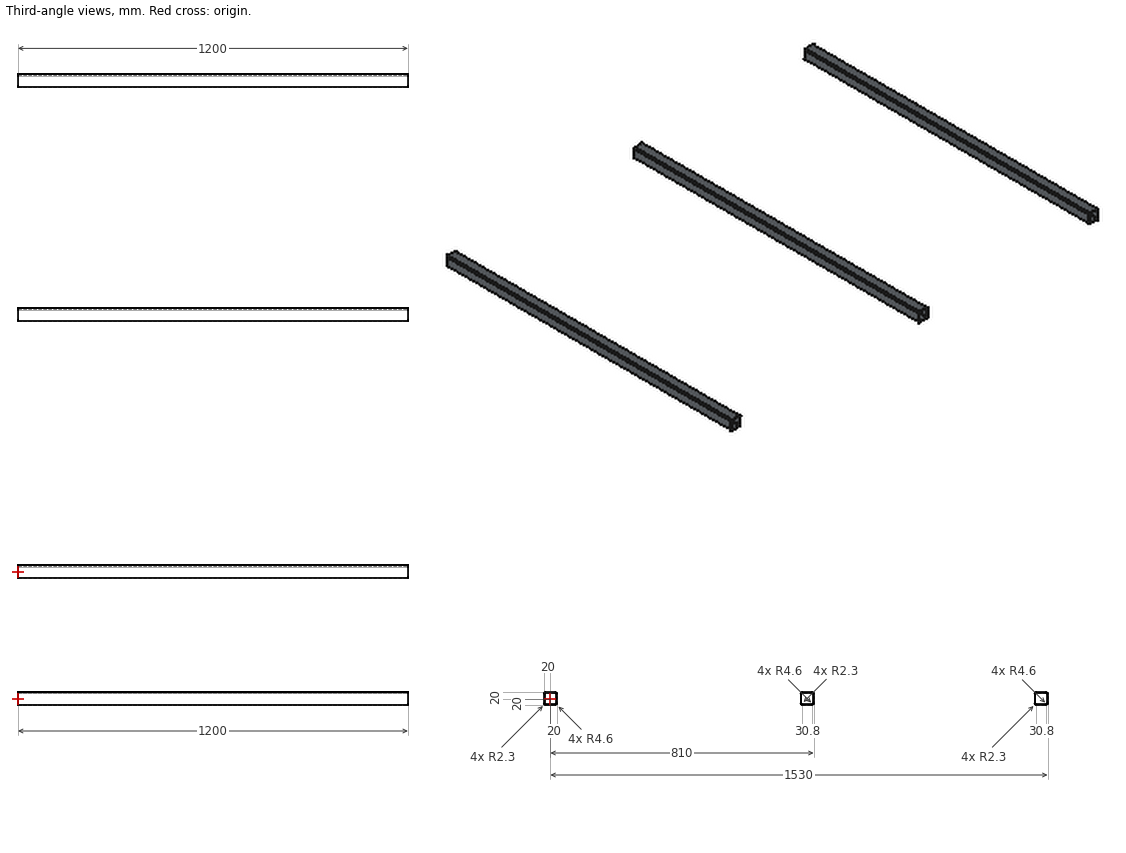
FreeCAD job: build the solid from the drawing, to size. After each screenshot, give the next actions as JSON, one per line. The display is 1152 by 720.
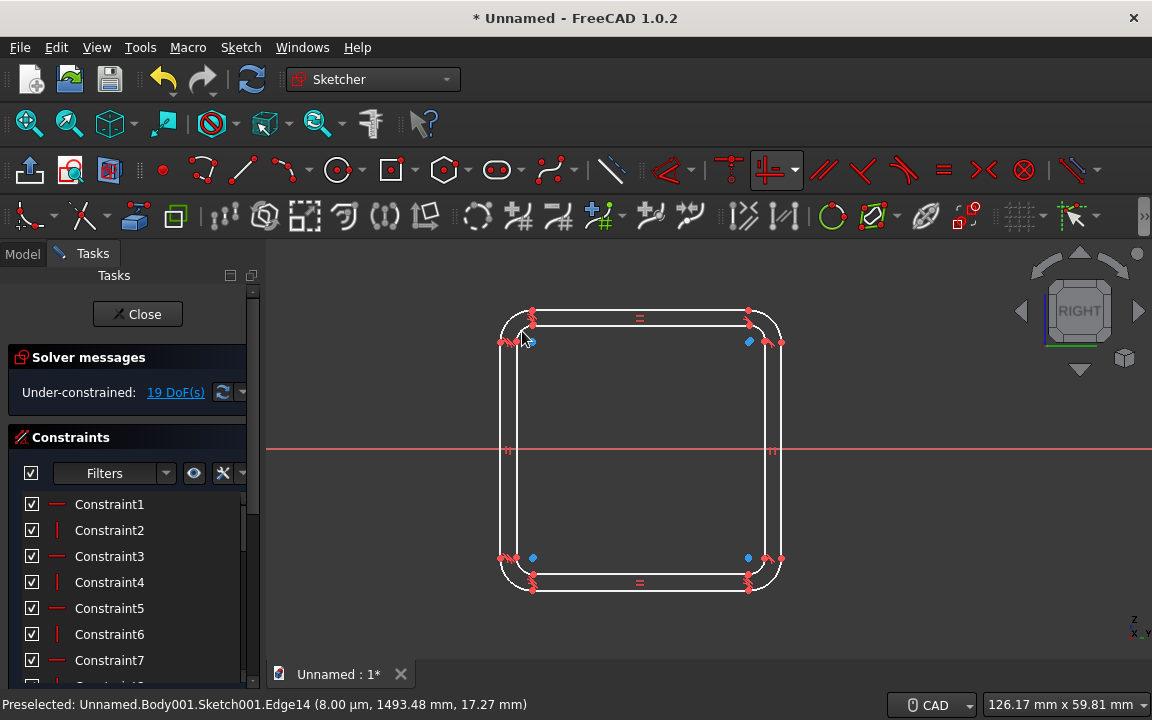
{"action": "left_click", "coordinate": [598, 326]}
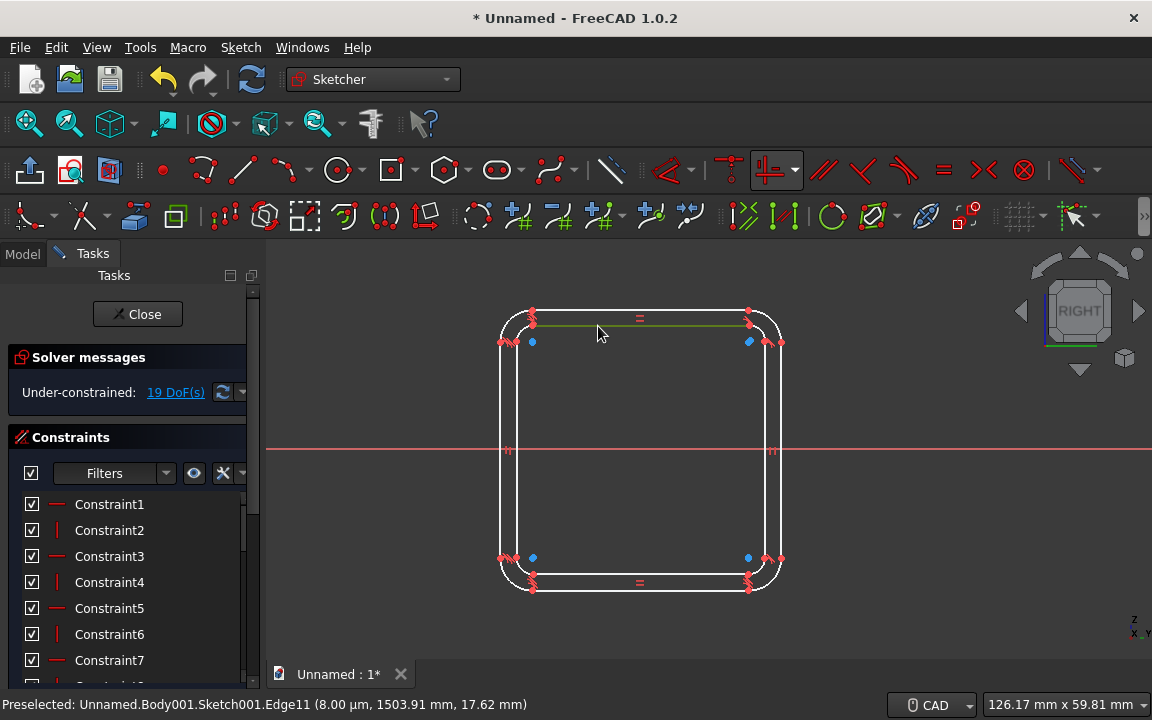
{"action": "left_click", "coordinate": [761, 330]}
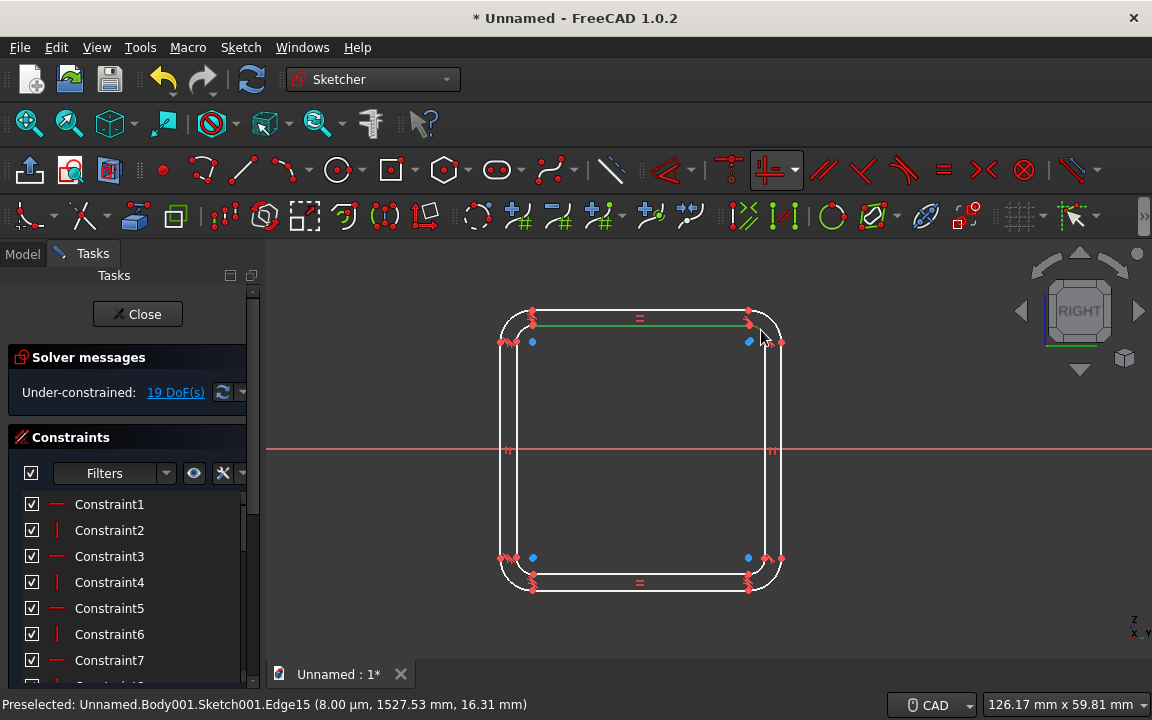
{"action": "key", "text": "t"}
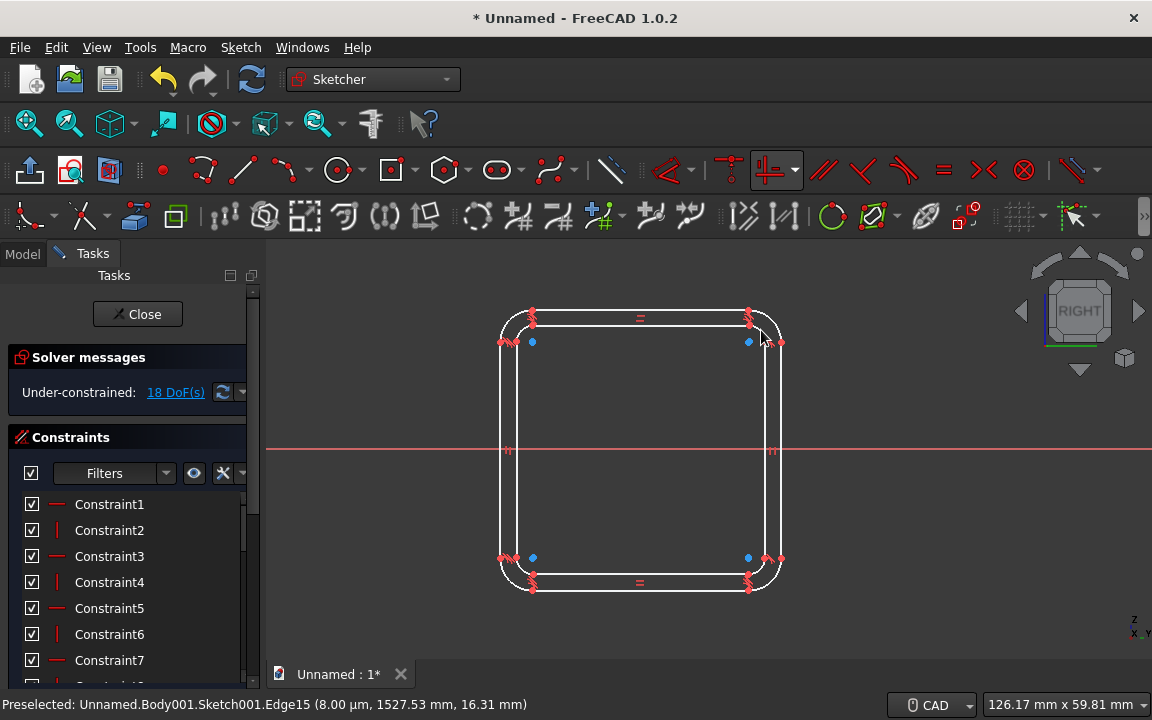
{"action": "left_click", "coordinate": [765, 407]}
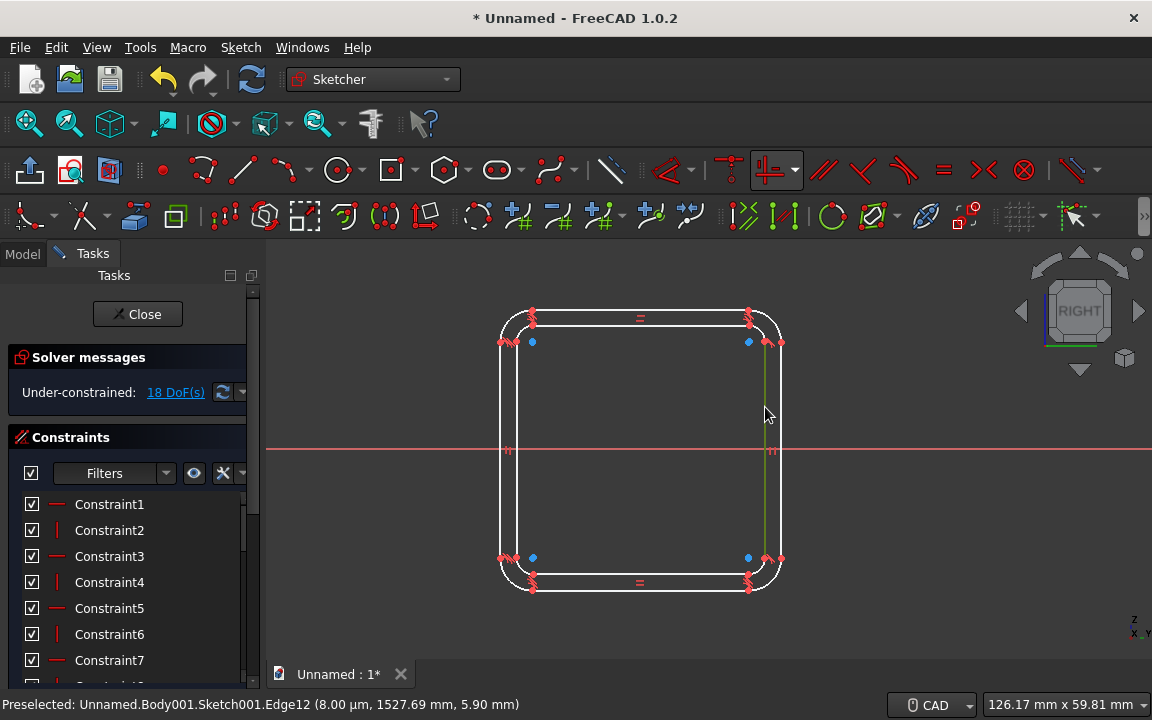
{"action": "left_click", "coordinate": [760, 330]}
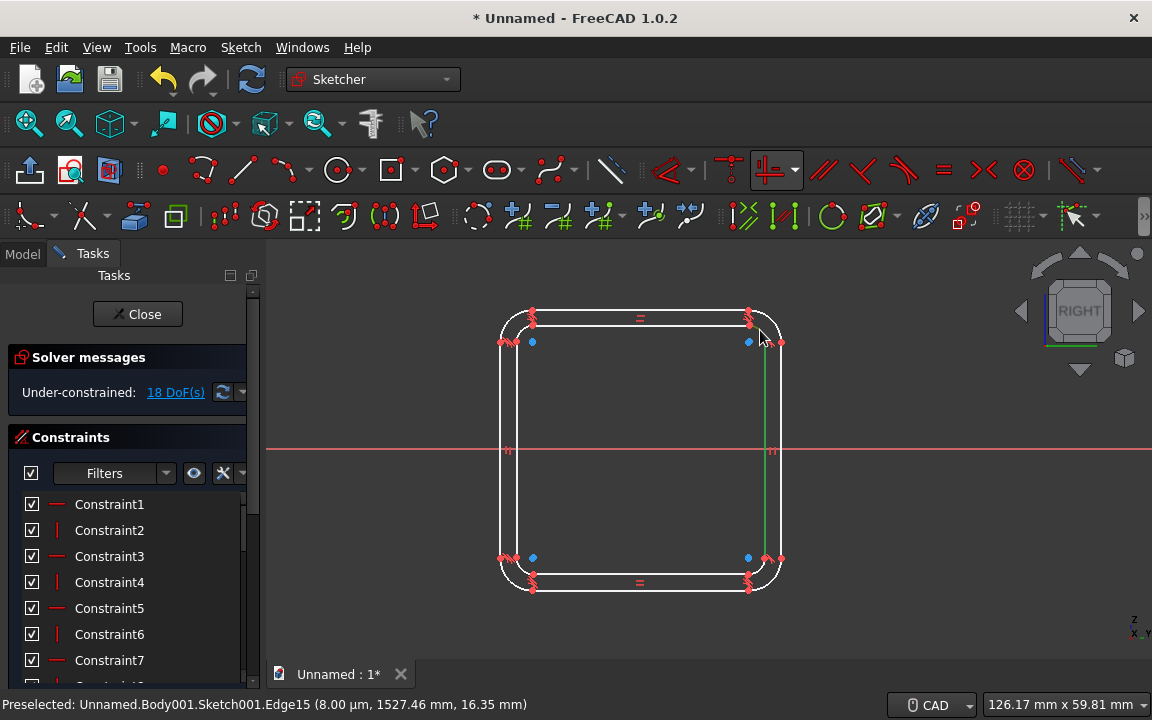
{"action": "left_click", "coordinate": [904, 170]}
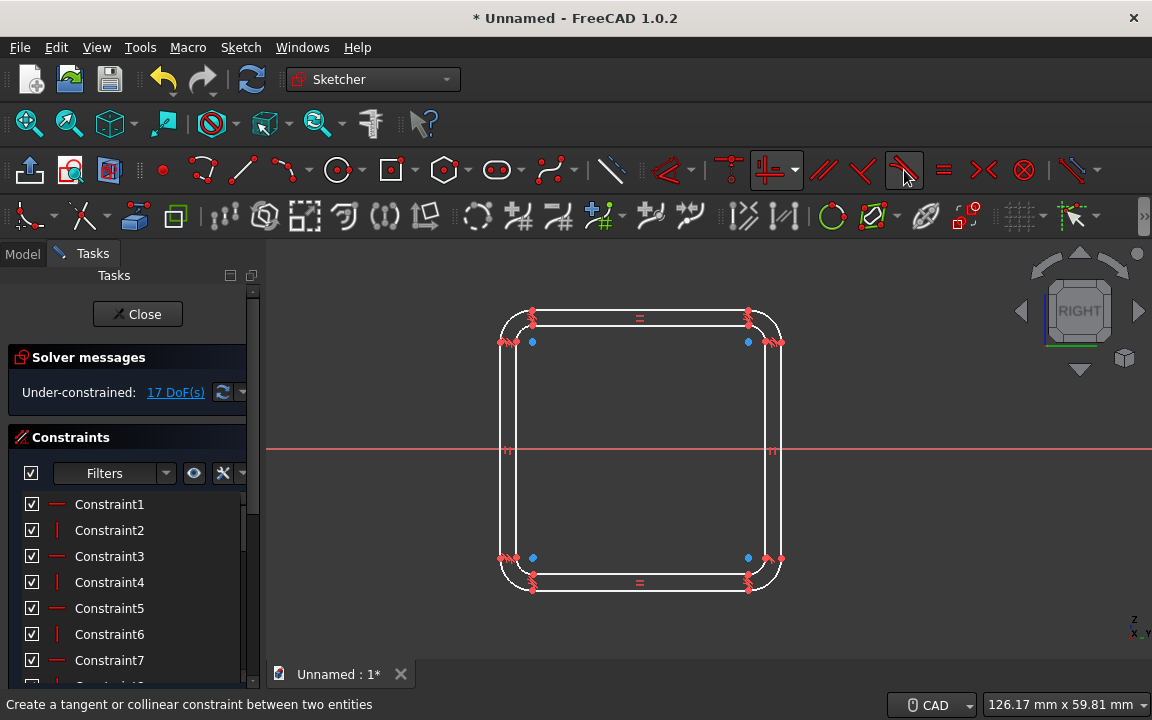
{"action": "left_click", "coordinate": [765, 407]}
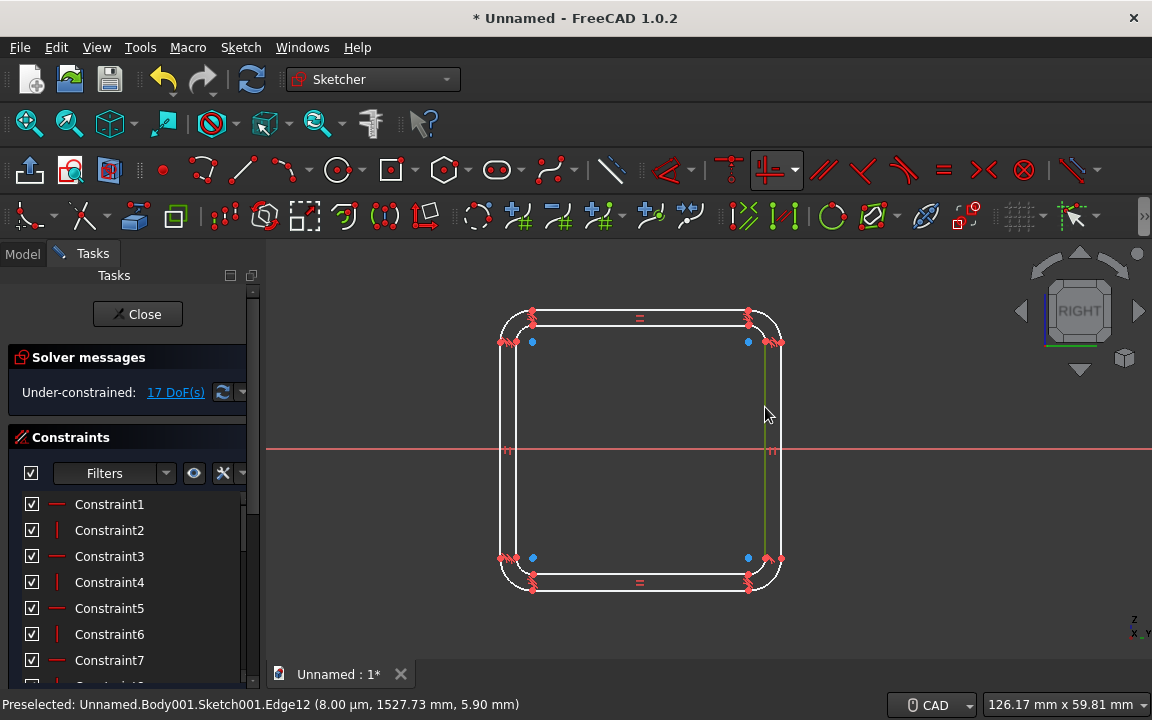
{"action": "left_click", "coordinate": [760, 570]}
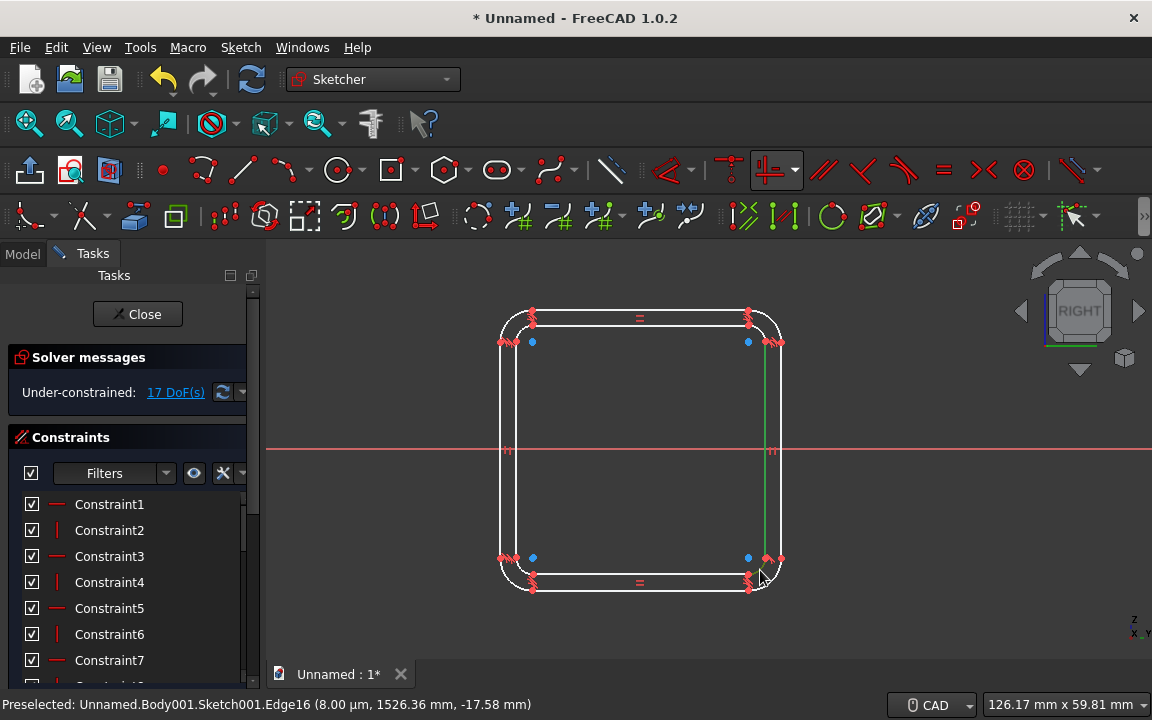
{"action": "key", "text": "t"}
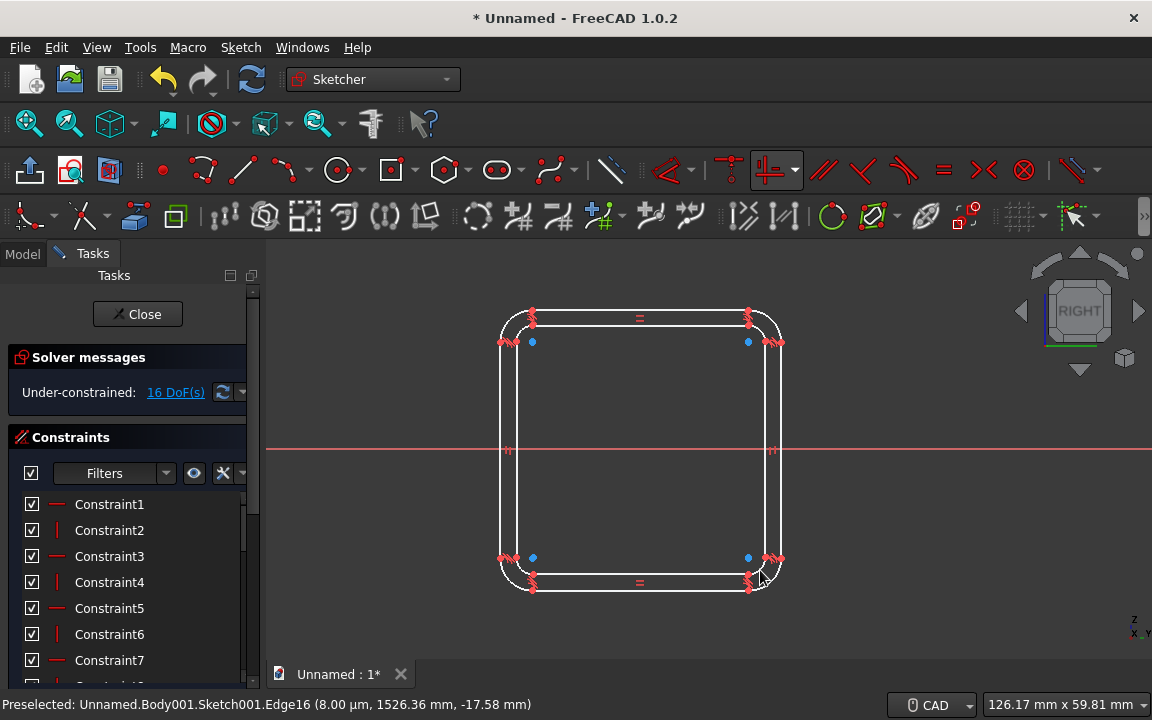
{"action": "left_click", "coordinate": [504, 573]}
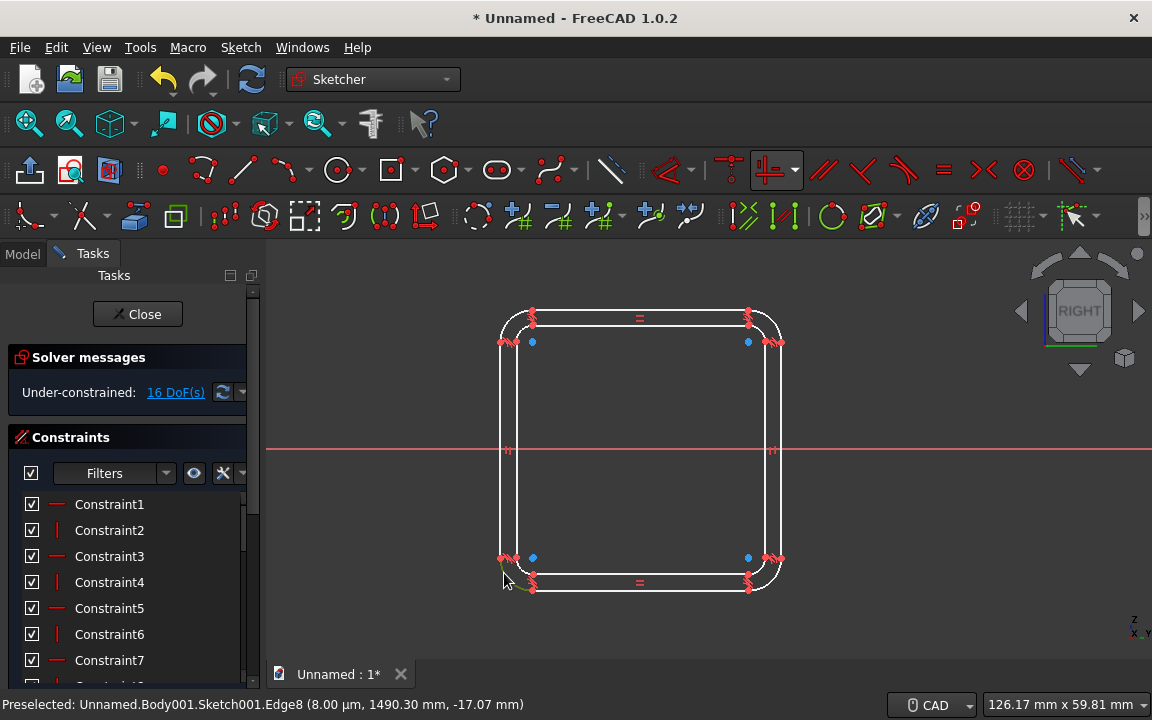
{"action": "left_click", "coordinate": [521, 570]}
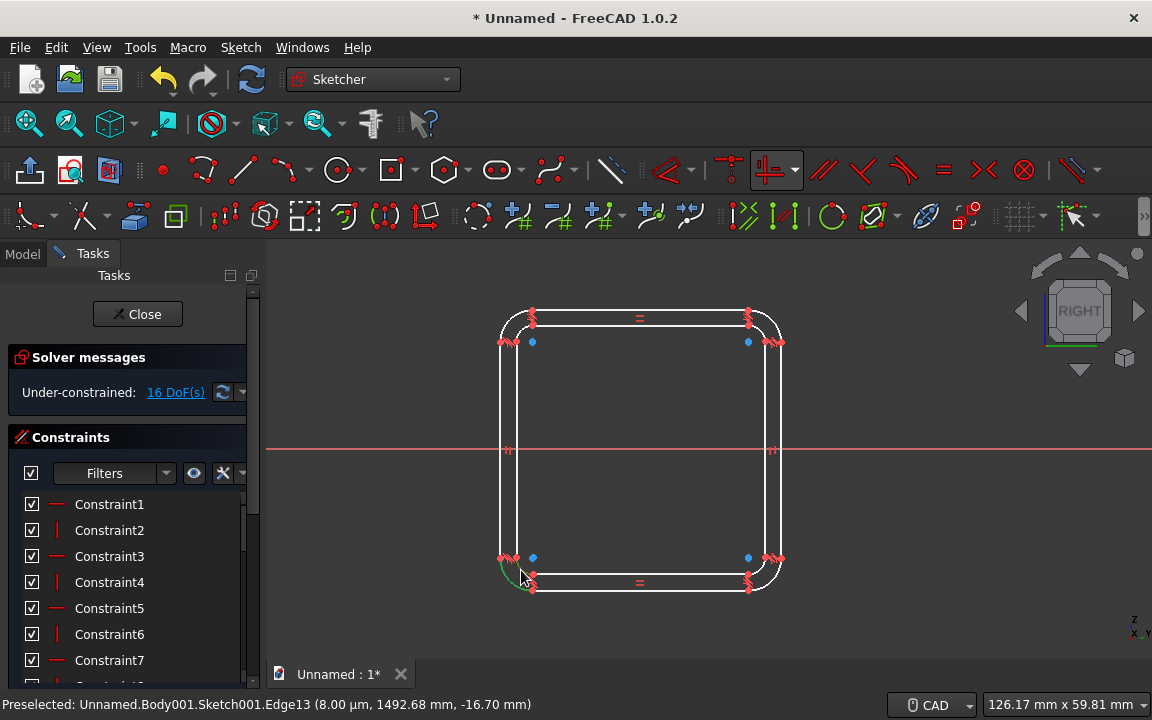
{"action": "key", "text": "c"}